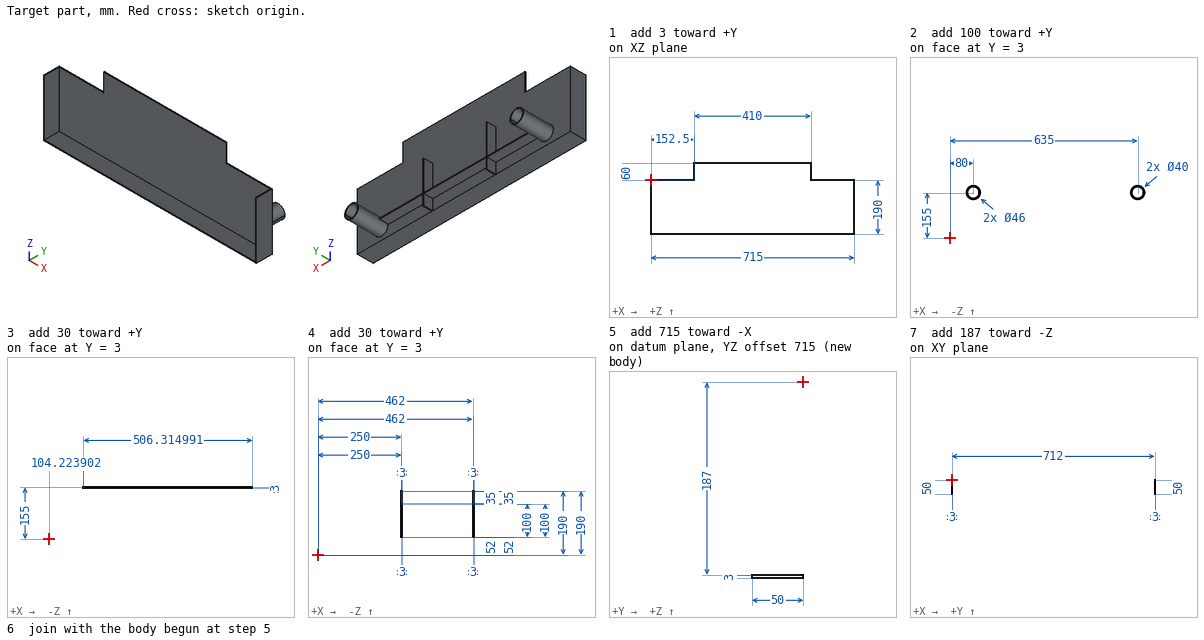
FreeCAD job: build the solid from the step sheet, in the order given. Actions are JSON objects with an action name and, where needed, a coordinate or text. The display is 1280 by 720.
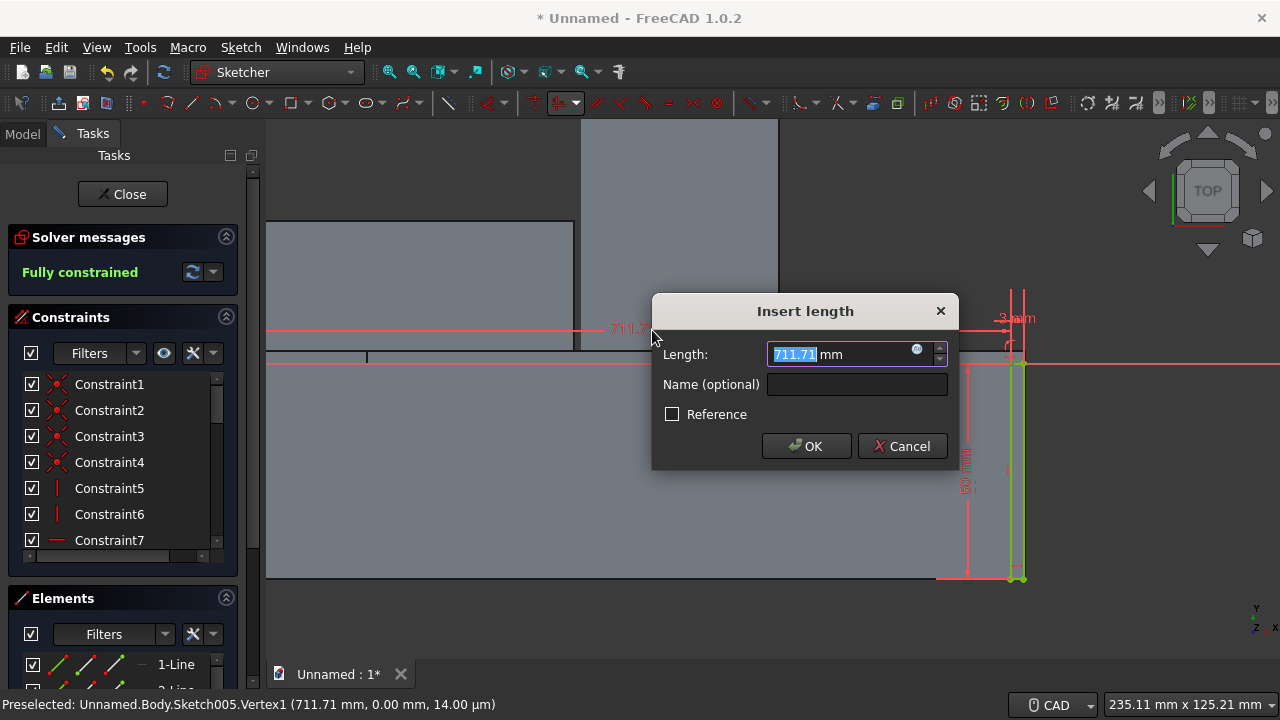
{"action": "type", "text": "712"}
{"action": "key", "text": "Return"}
{"action": "key", "text": "Escape"}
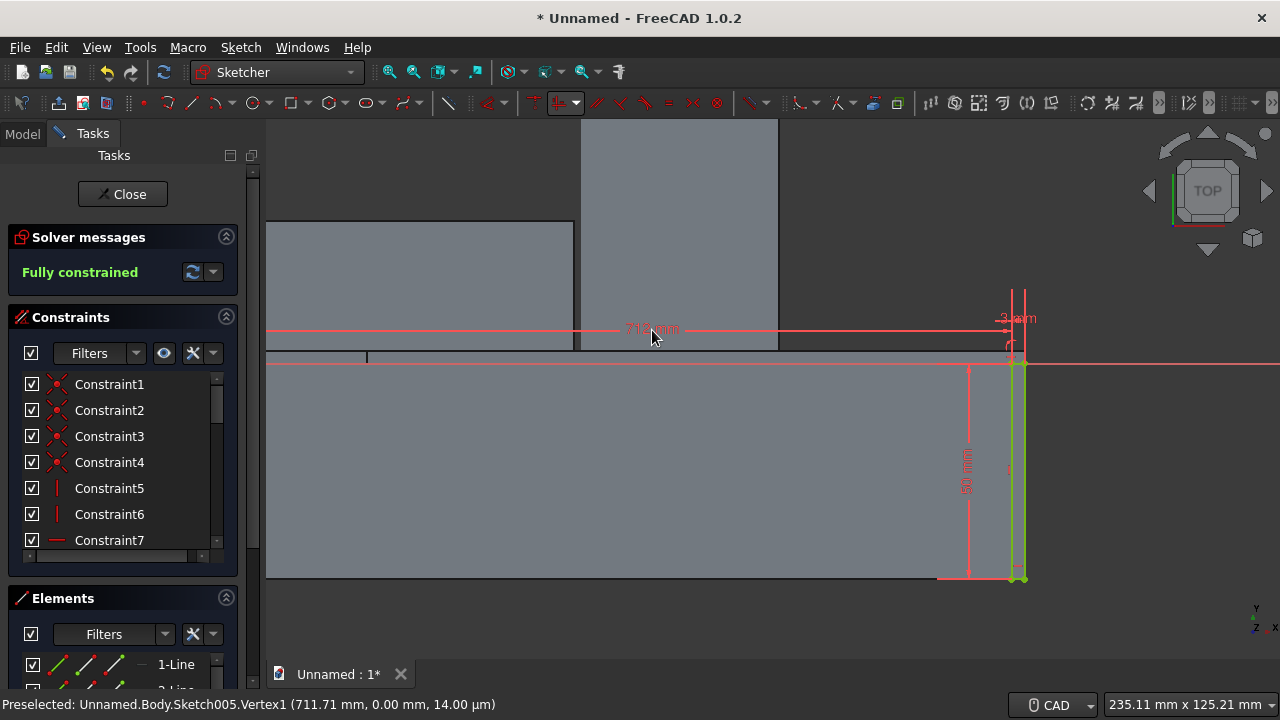
{"action": "left_click", "coordinate": [123, 194]}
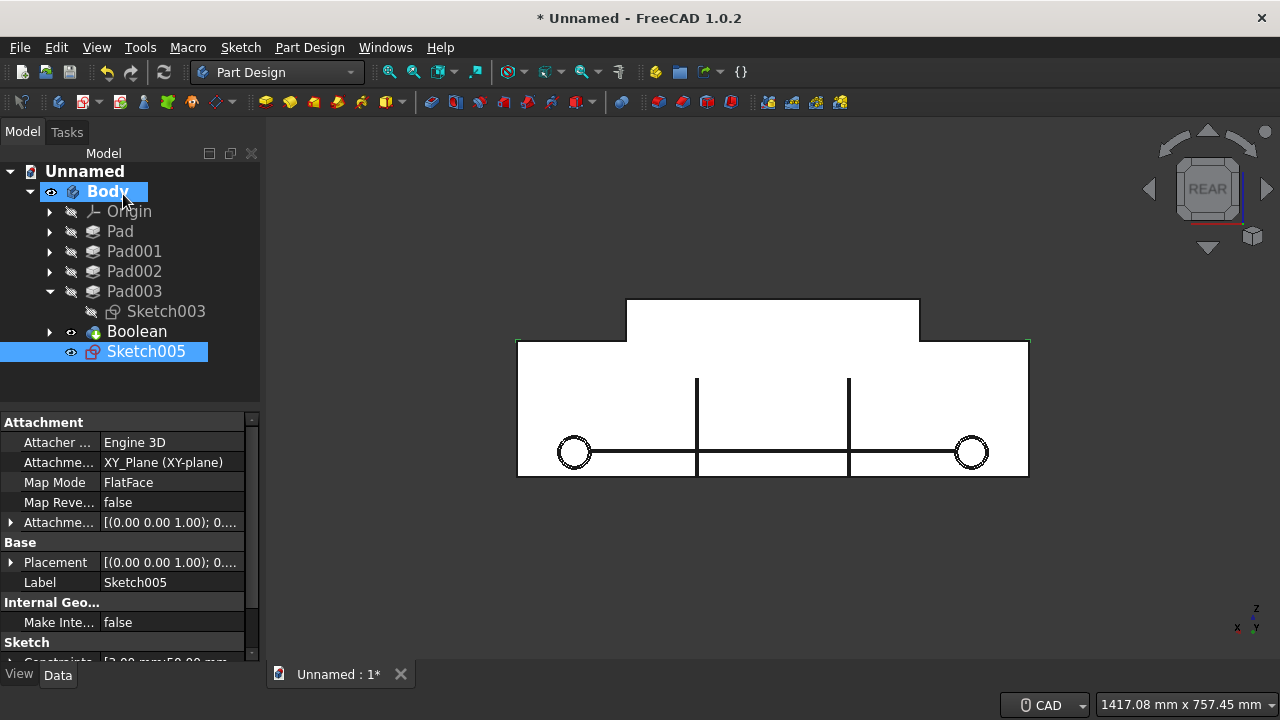
{"action": "left_click", "coordinate": [266, 102]}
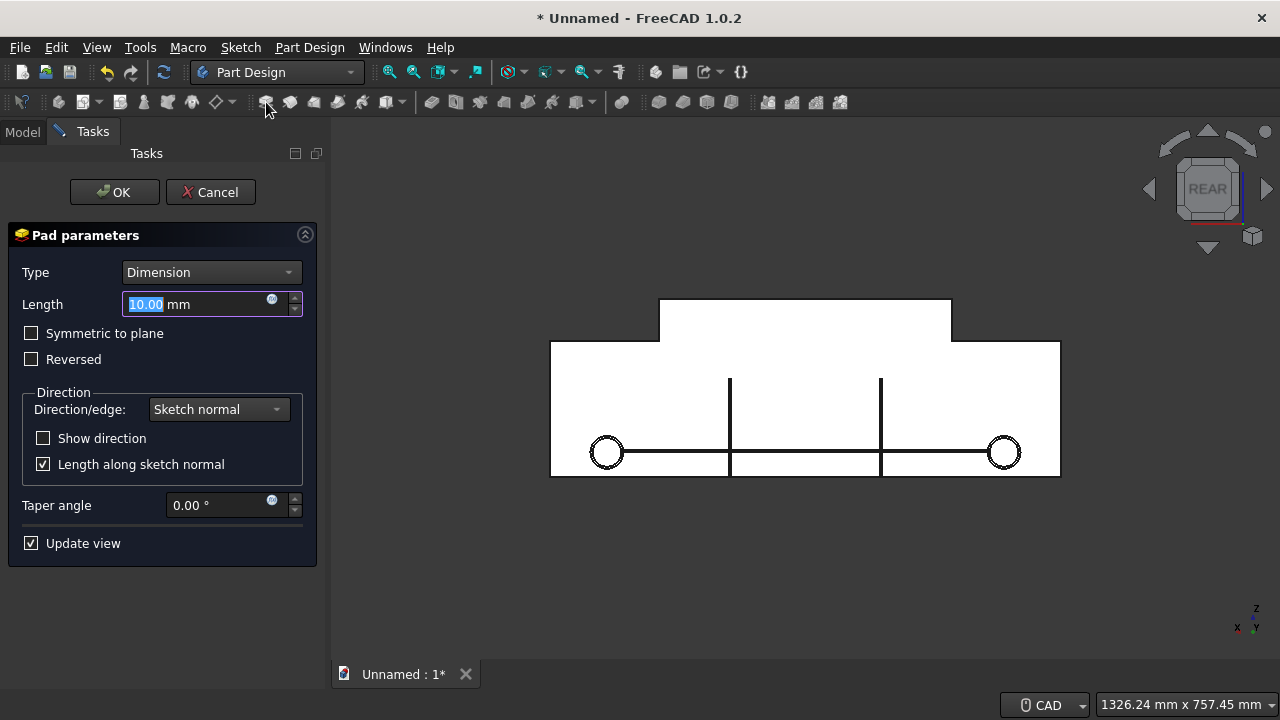
{"action": "type", "text": "187"}
{"action": "key", "text": "Tab"}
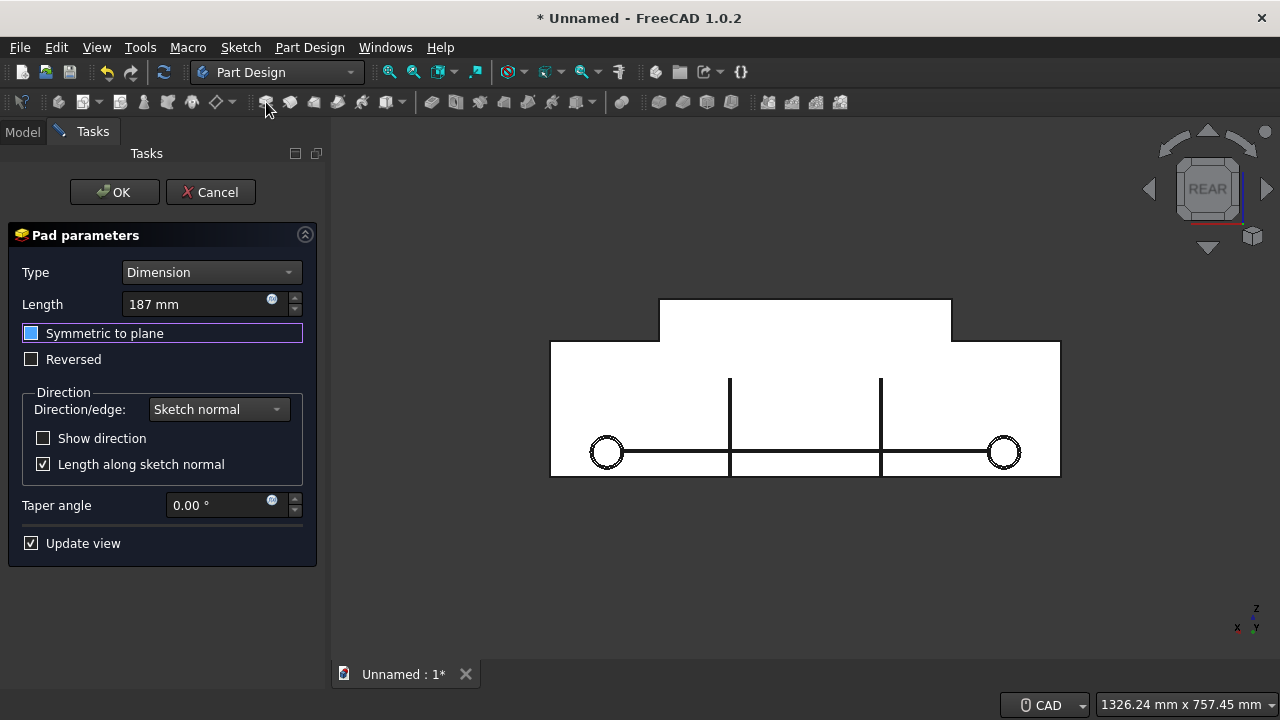
{"action": "left_click", "coordinate": [30, 359]}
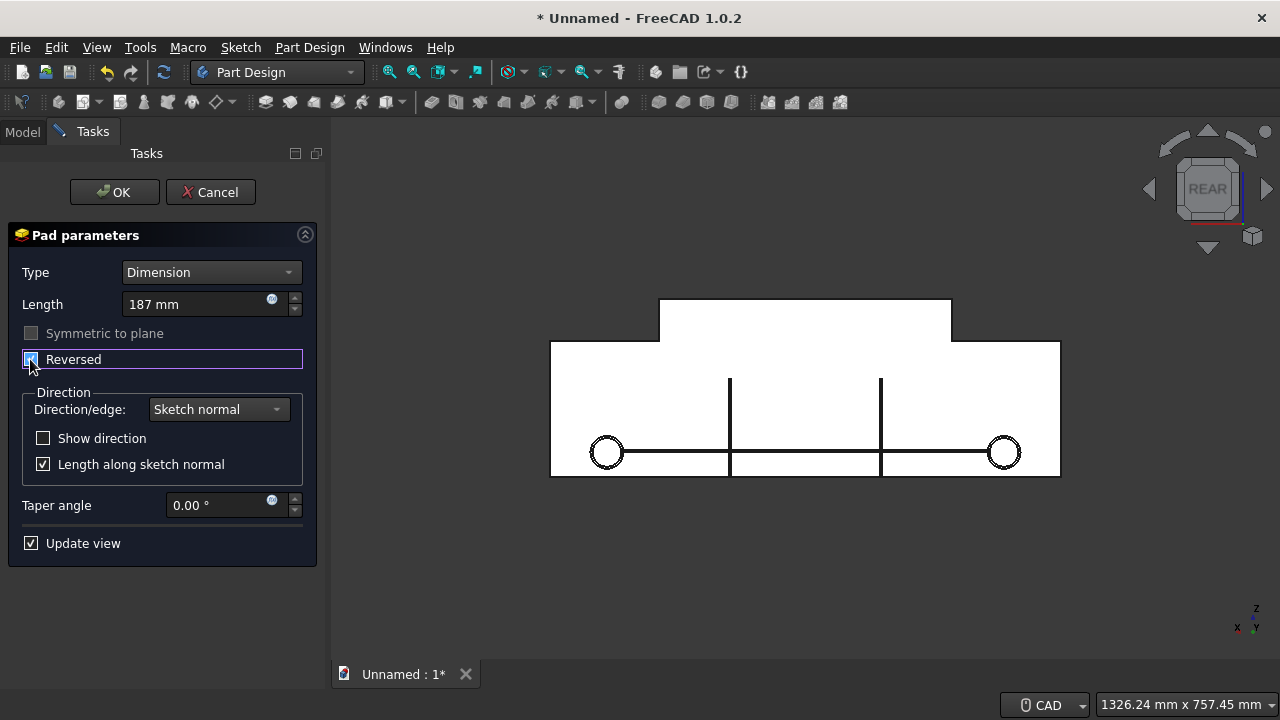
{"action": "left_click", "coordinate": [115, 192]}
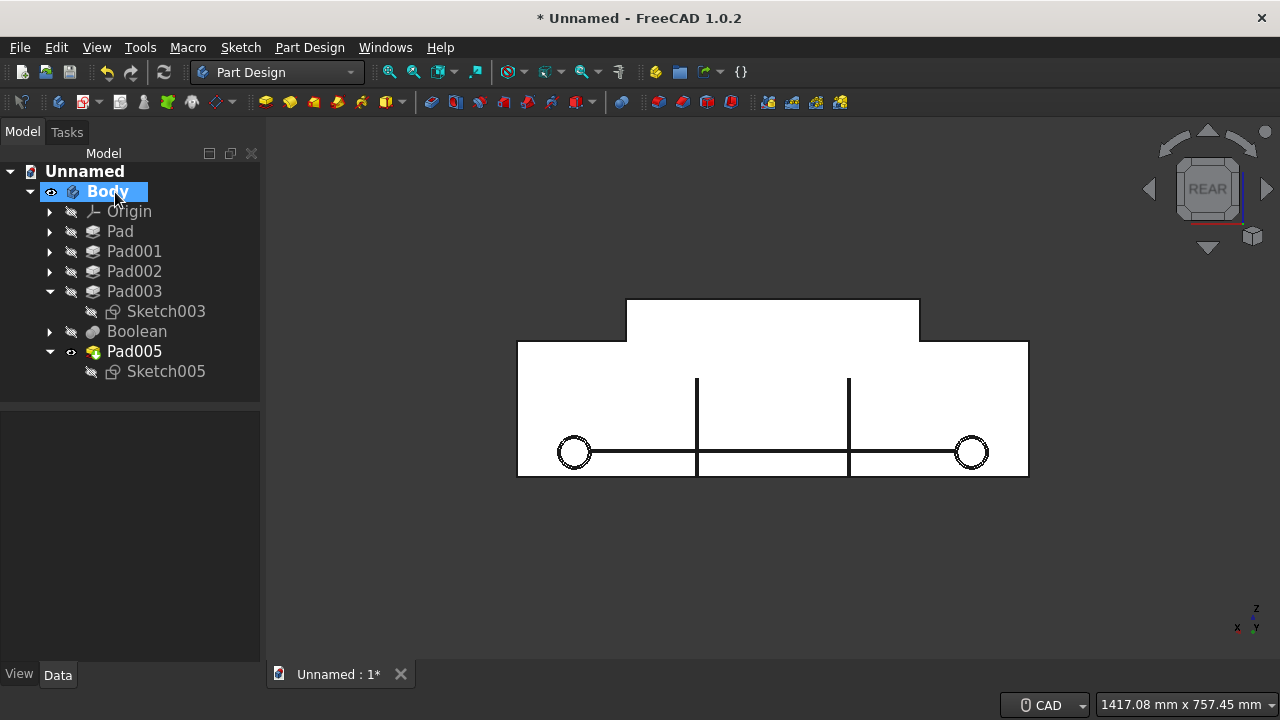
{"action": "key", "text": "0"}